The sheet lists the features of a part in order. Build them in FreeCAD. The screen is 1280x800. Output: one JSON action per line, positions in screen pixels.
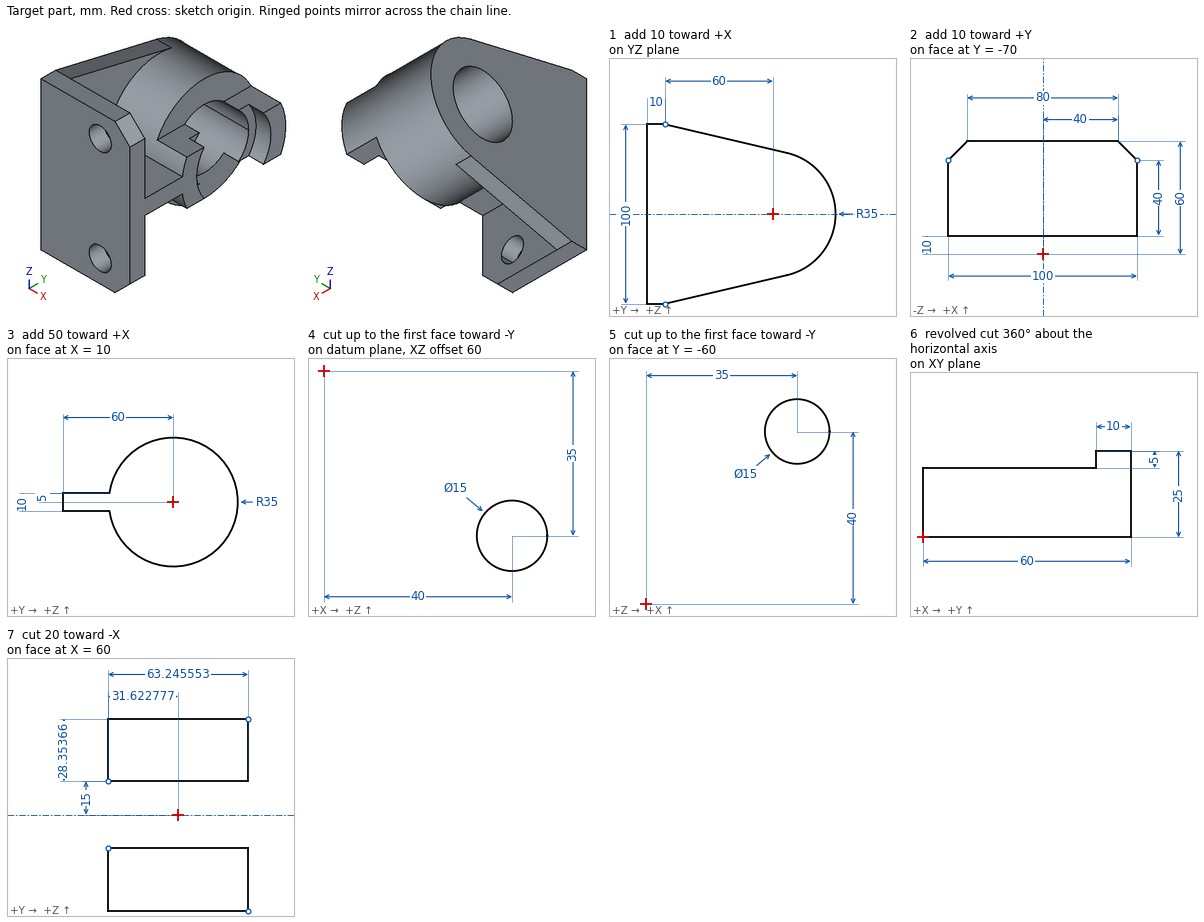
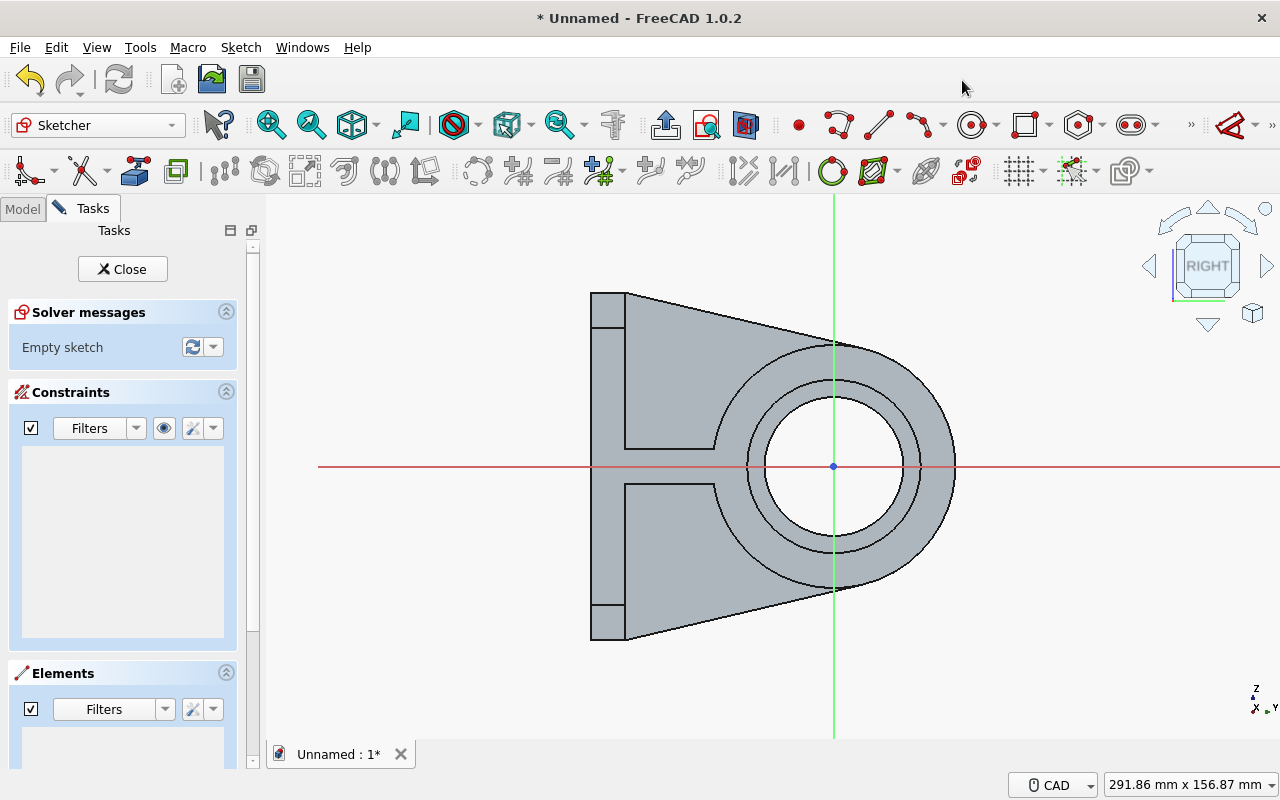
{"action": "left_click", "coordinate": [1026, 126]}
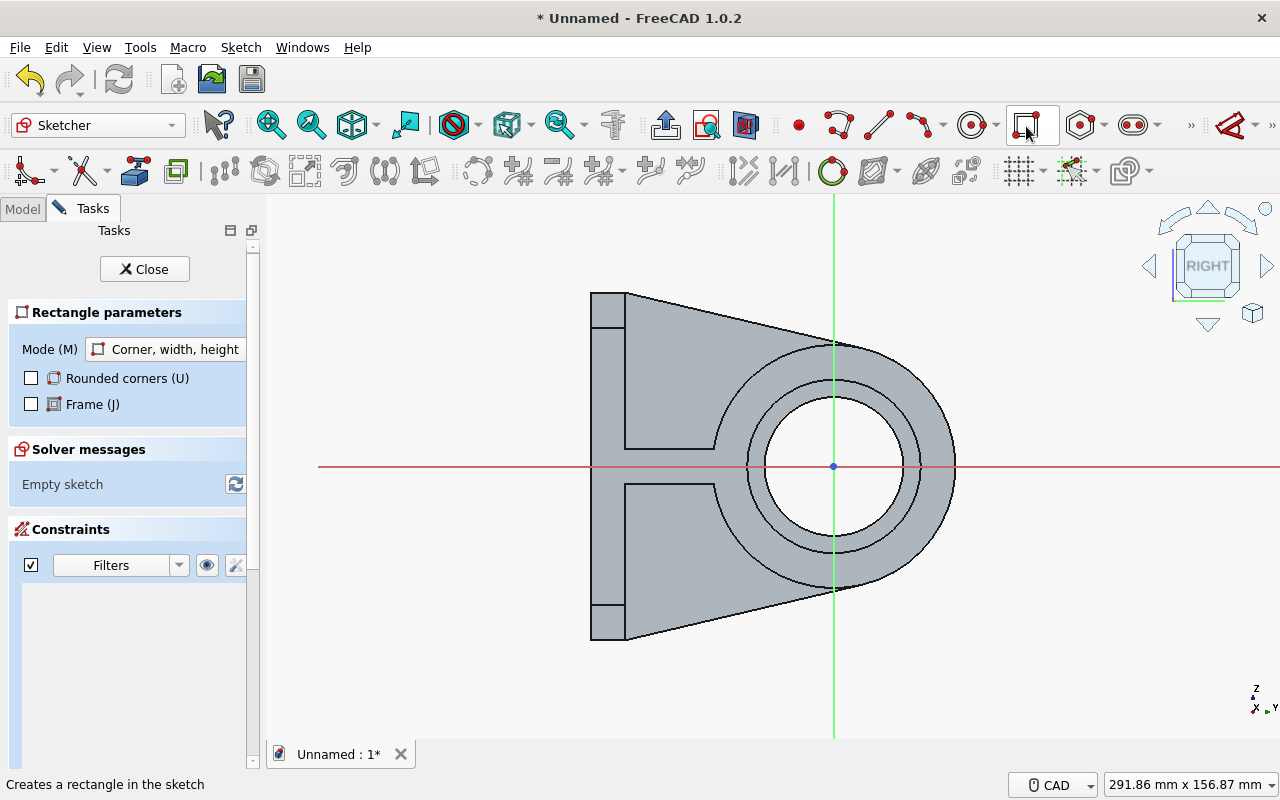
{"action": "left_click", "coordinate": [724, 316]}
{"action": "left_click", "coordinate": [944, 414]}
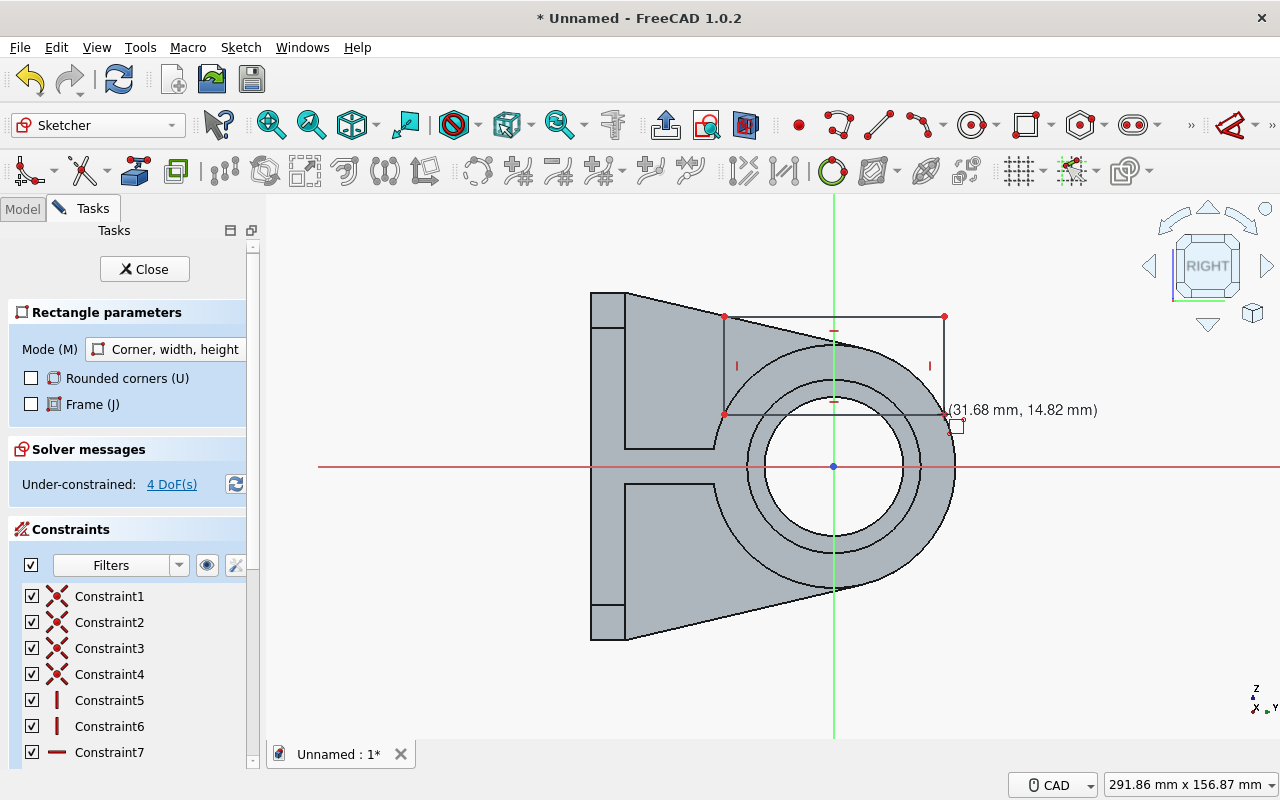
{"action": "left_click", "coordinate": [724, 519]}
{"action": "left_click", "coordinate": [944, 617]}
{"action": "key", "text": "Escape"}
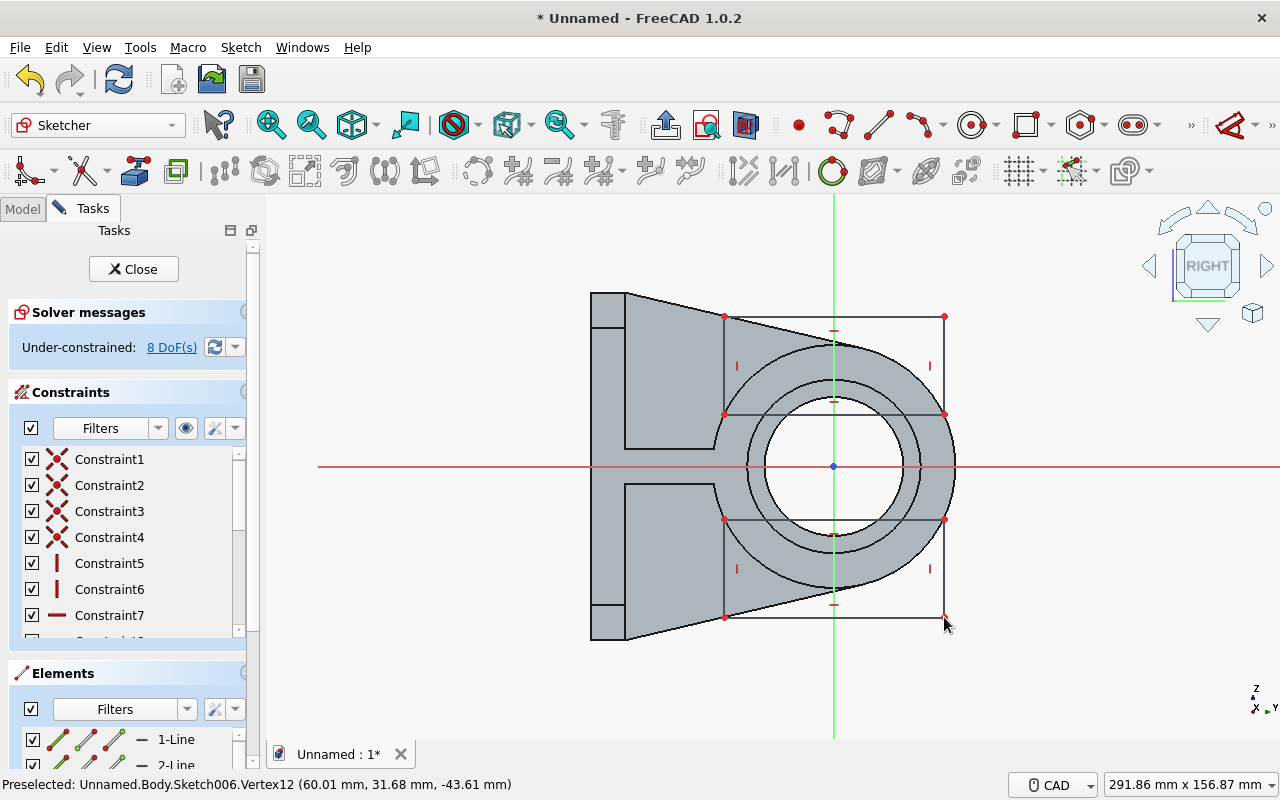
{"action": "left_click", "coordinate": [724, 415]}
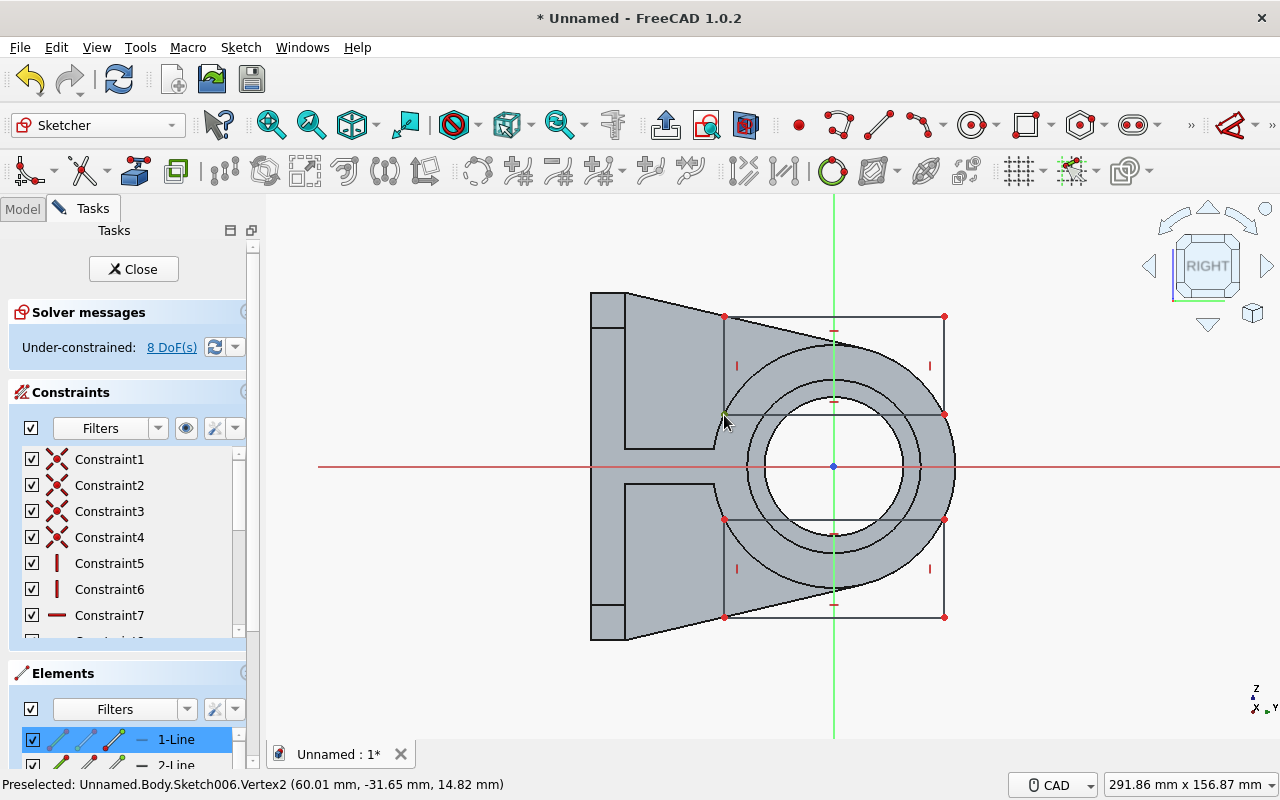
{"action": "left_click", "coordinate": [724, 520]}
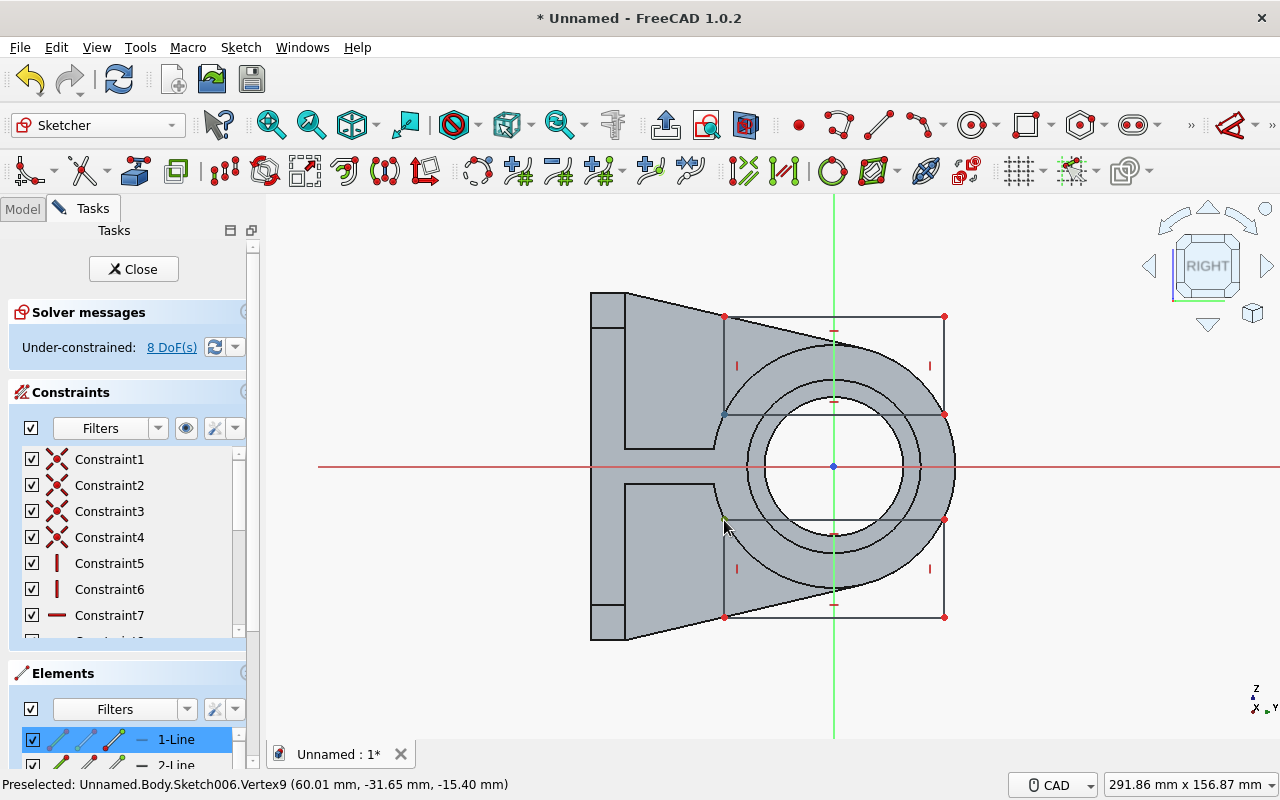
{"action": "left_click", "coordinate": [353, 466]}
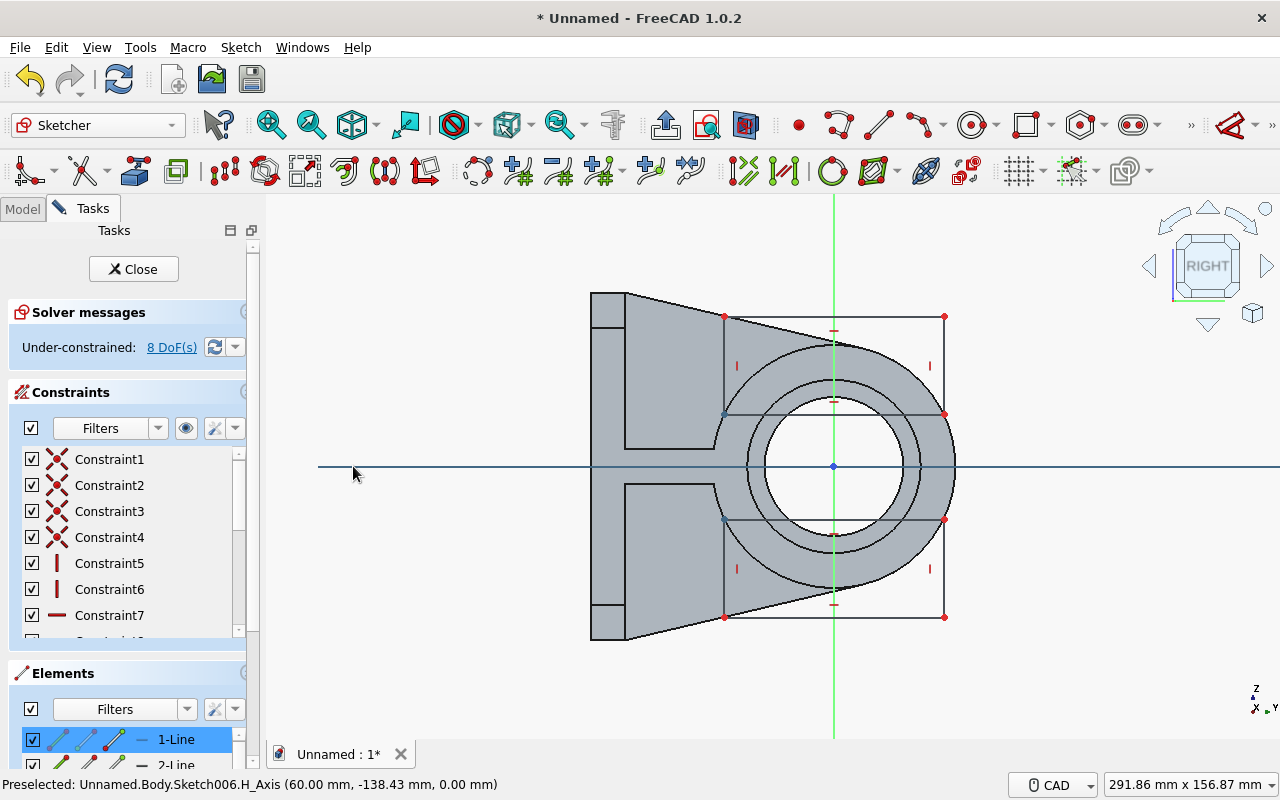
{"action": "key", "text": "s"}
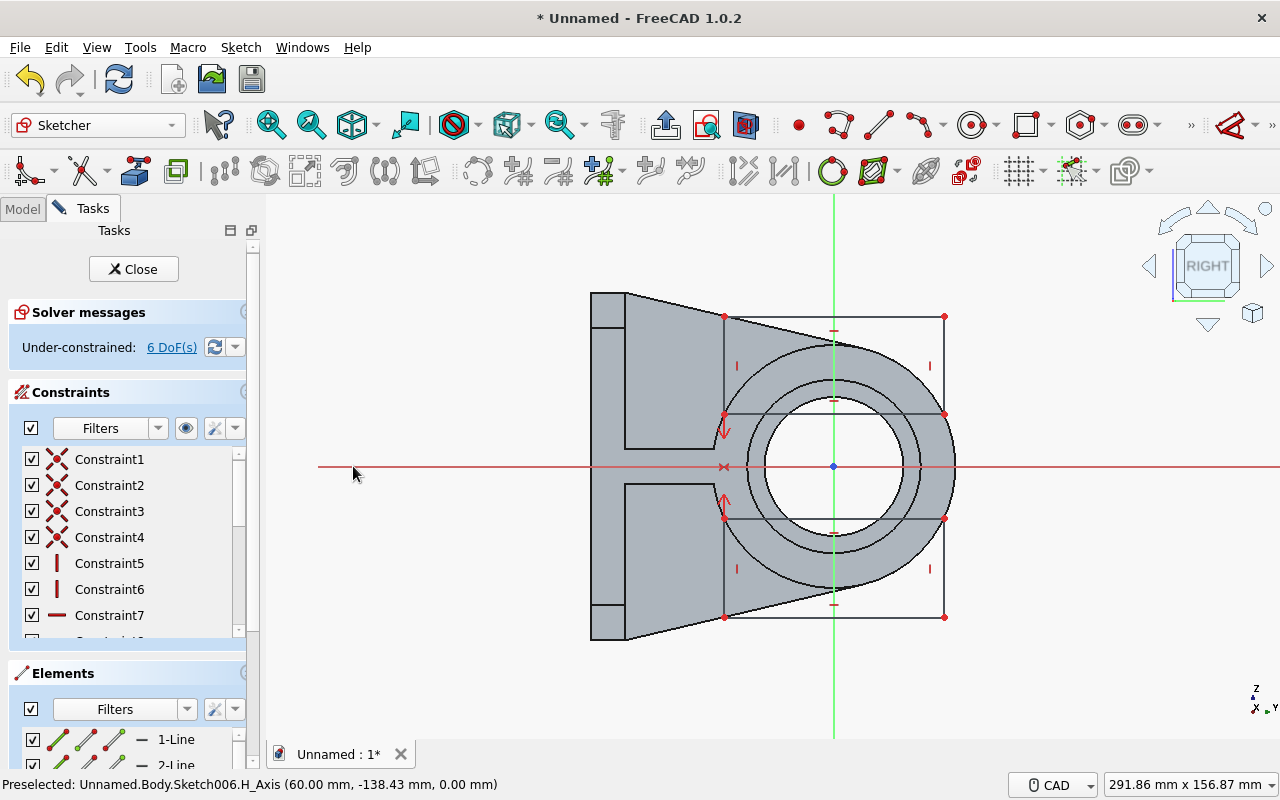
{"action": "left_click", "coordinate": [944, 317]}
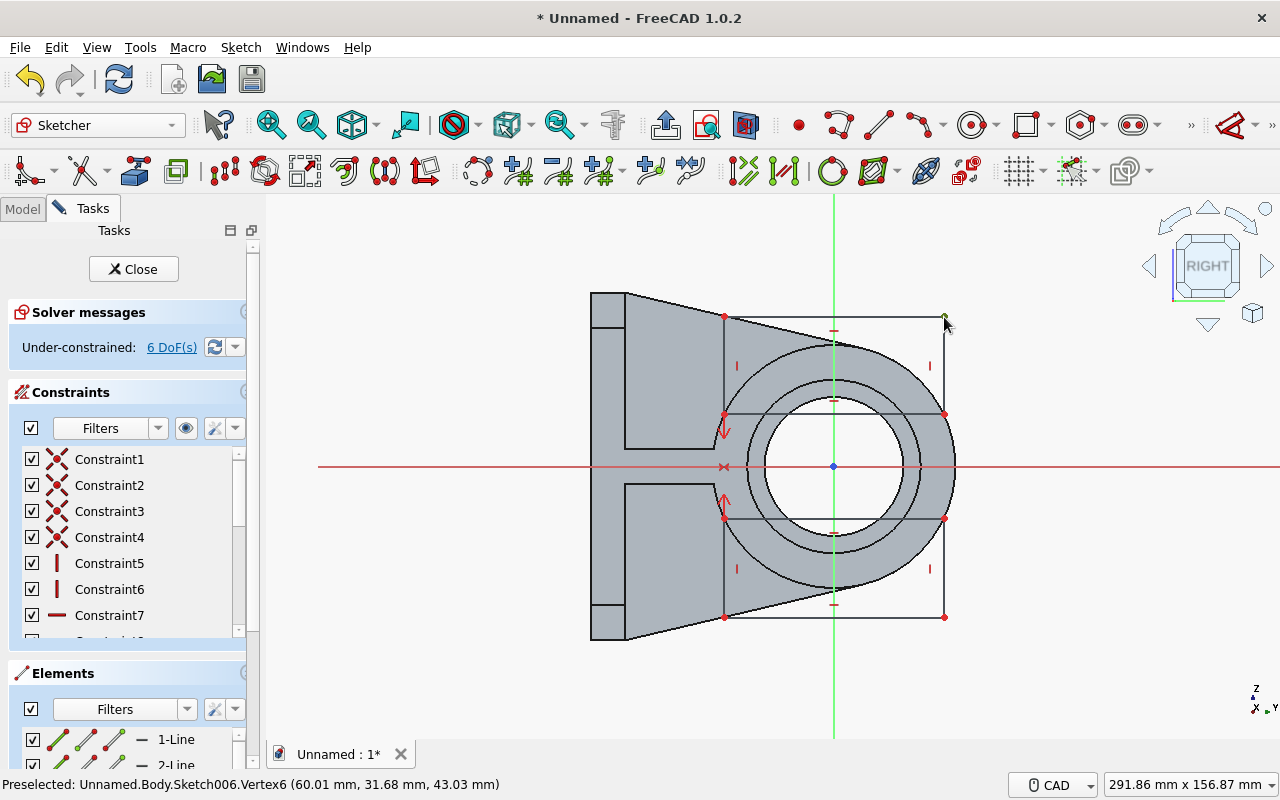
{"action": "left_click", "coordinate": [944, 618]}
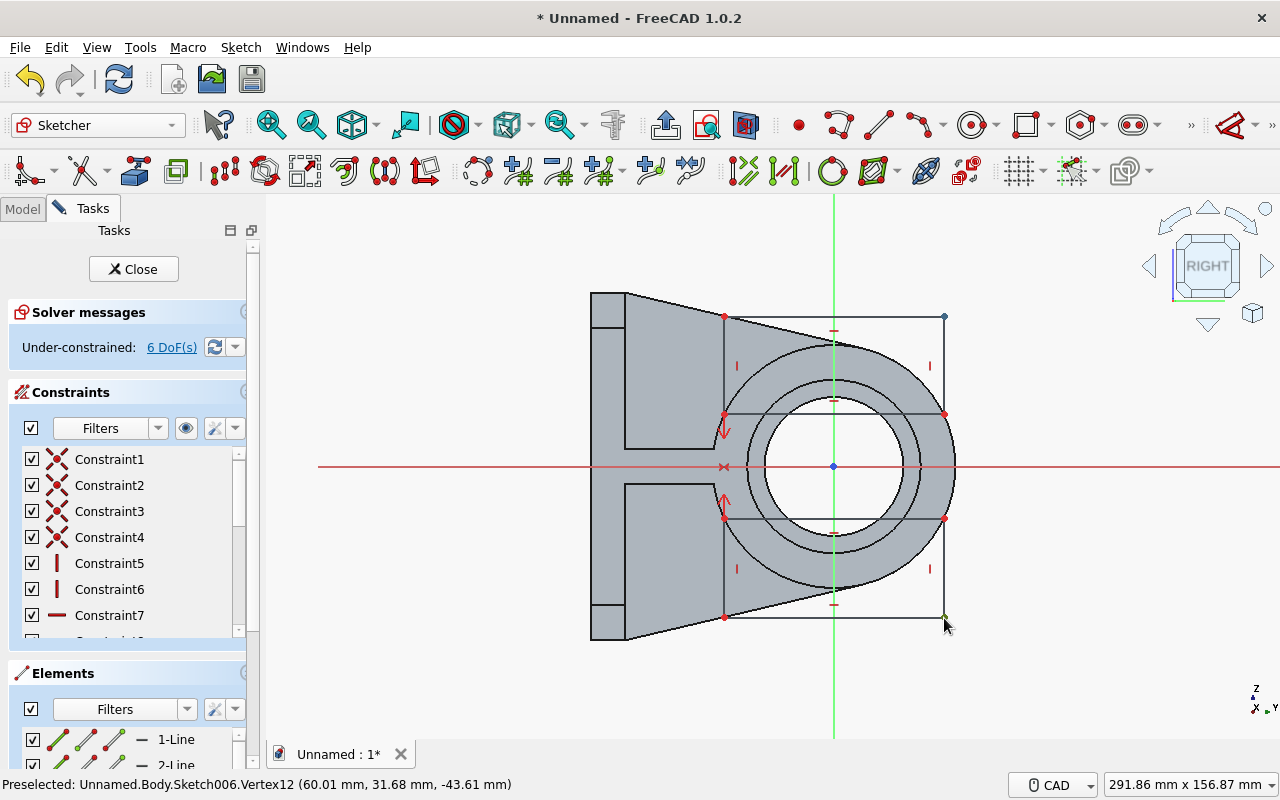
{"action": "left_click", "coordinate": [353, 466]}